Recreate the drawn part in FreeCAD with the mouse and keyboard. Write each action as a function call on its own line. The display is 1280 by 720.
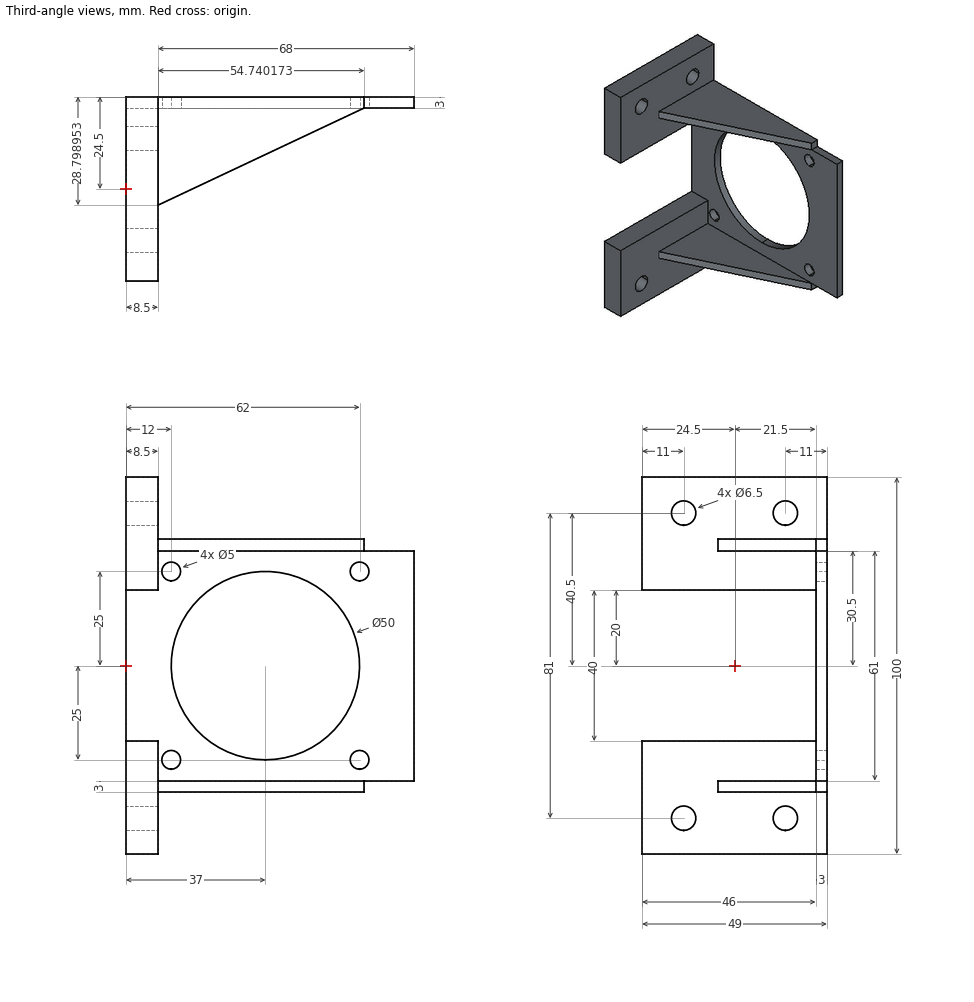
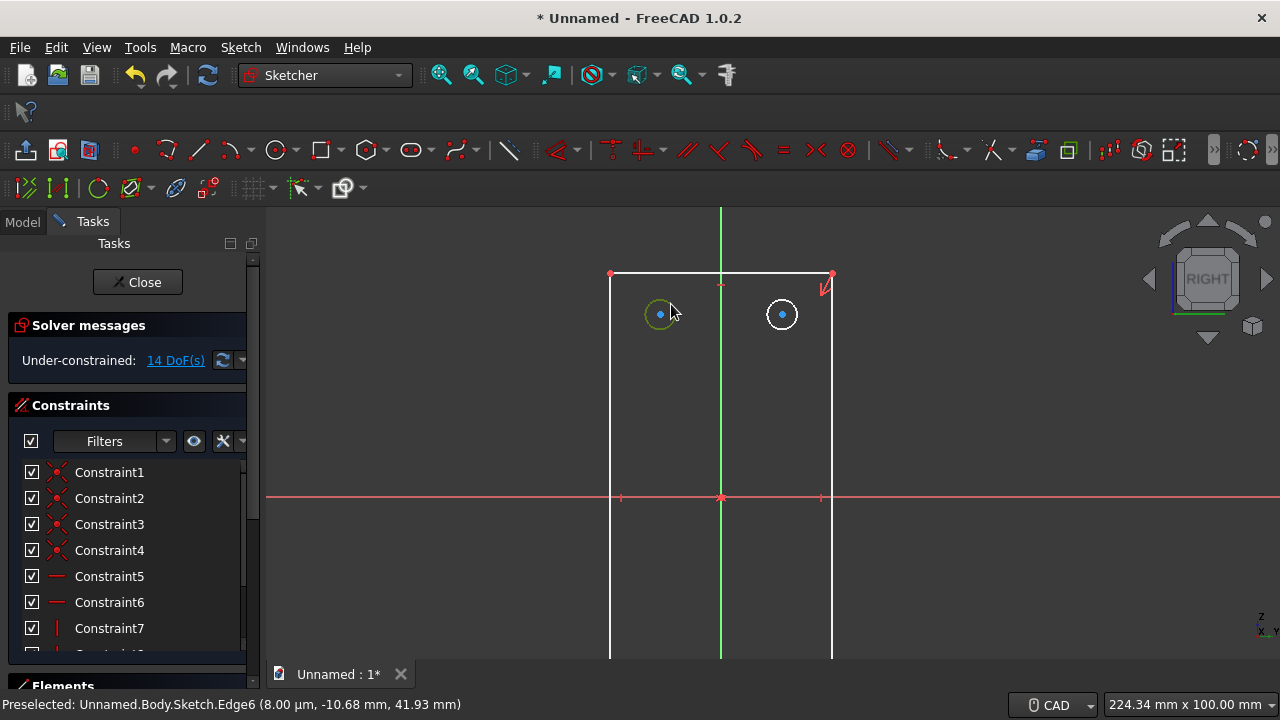
scroll(670, 303, down, 2)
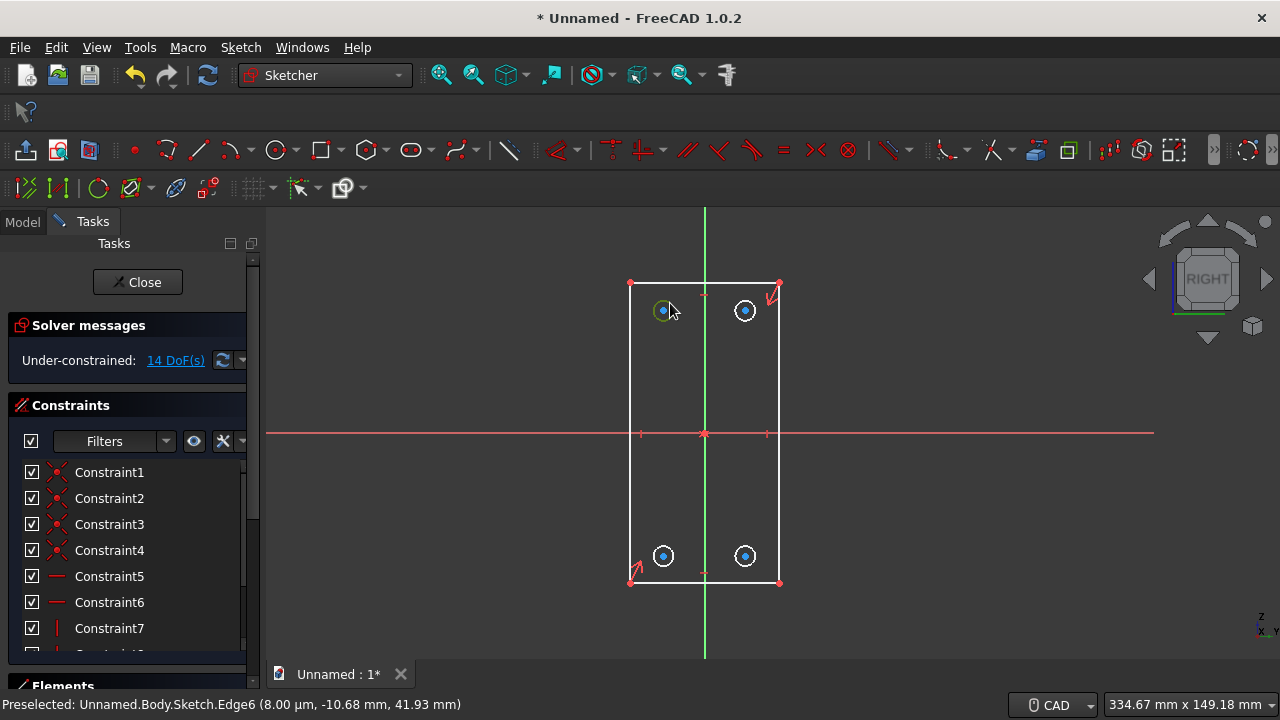
scroll(670, 549, up, 2)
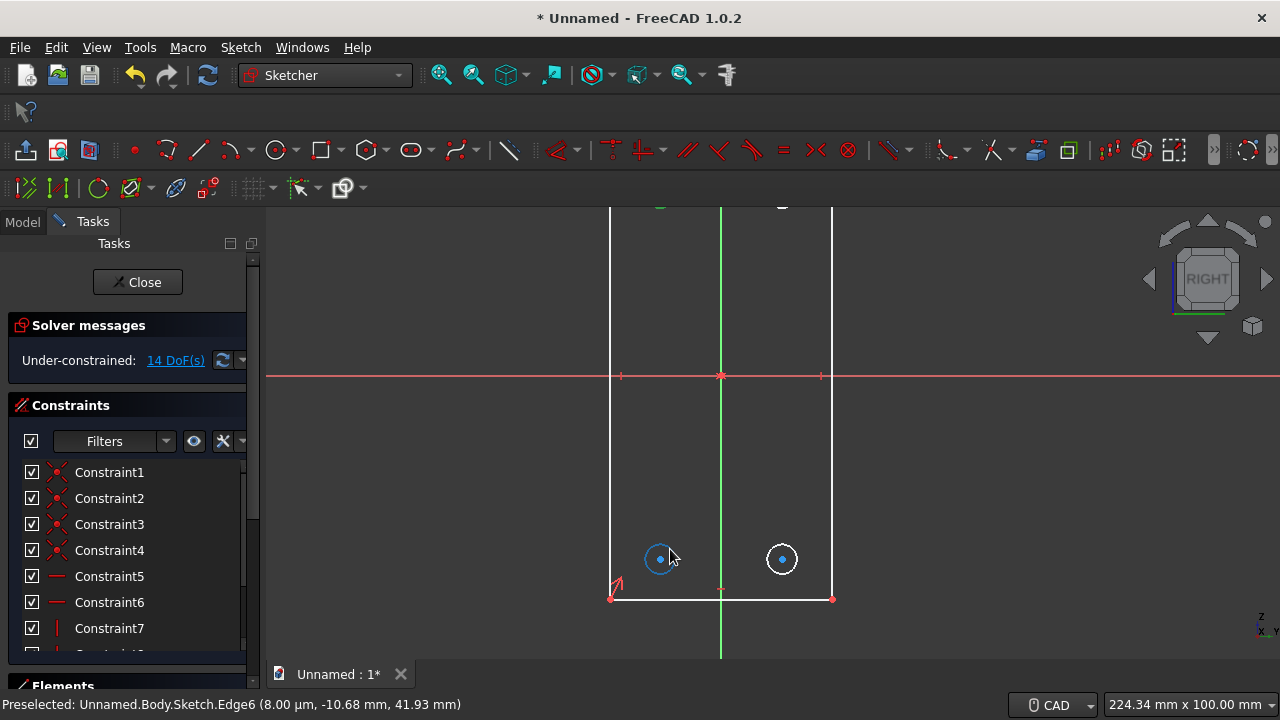
click(671, 549)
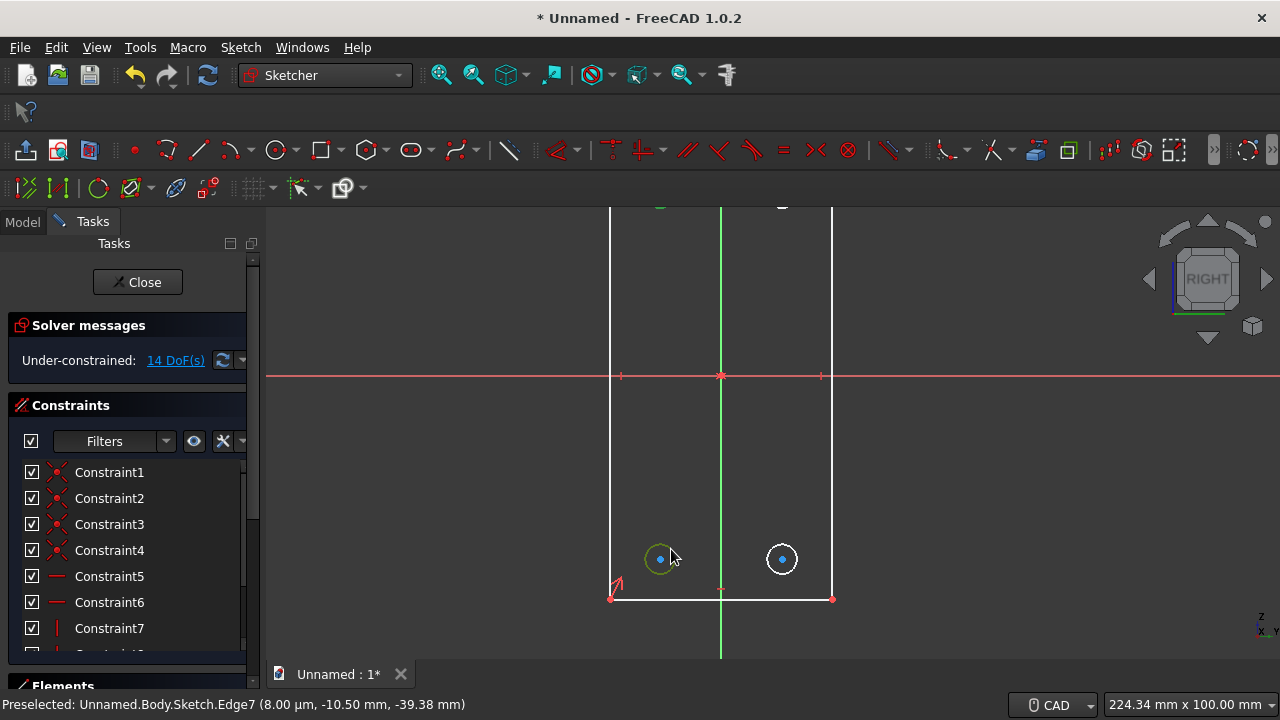
scroll(670, 549, down, 2)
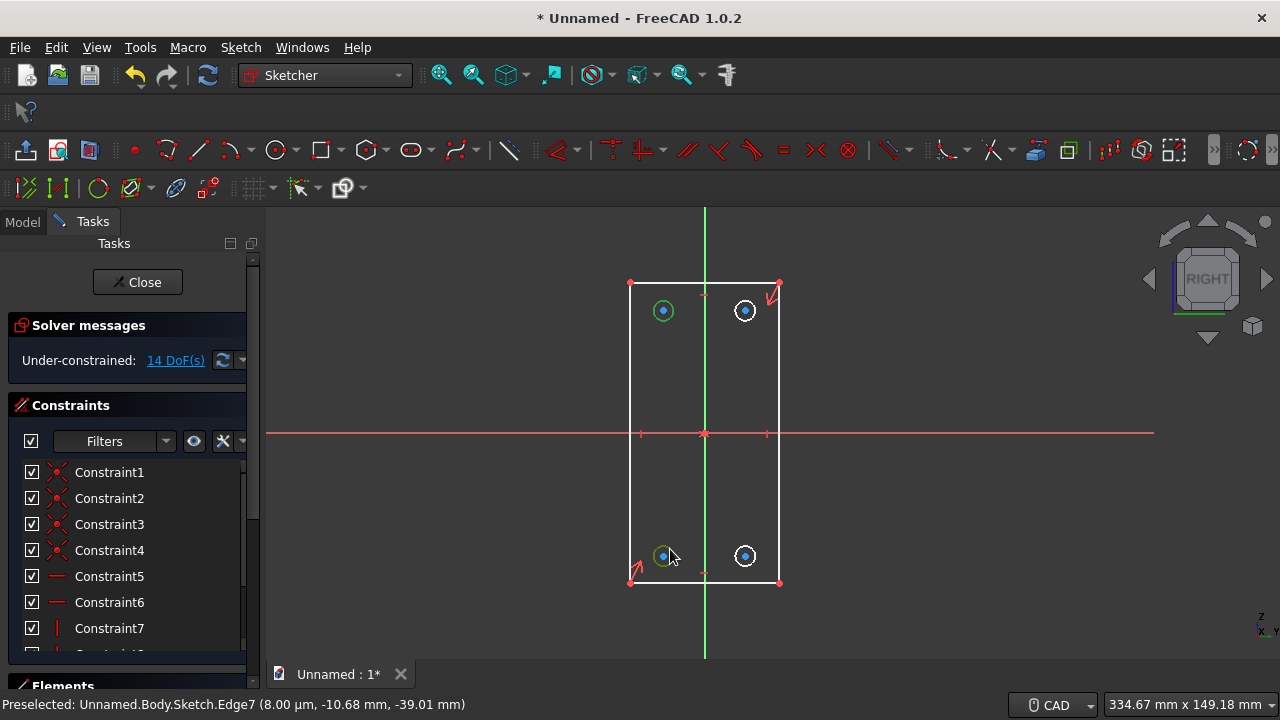
scroll(752, 304, up, 2)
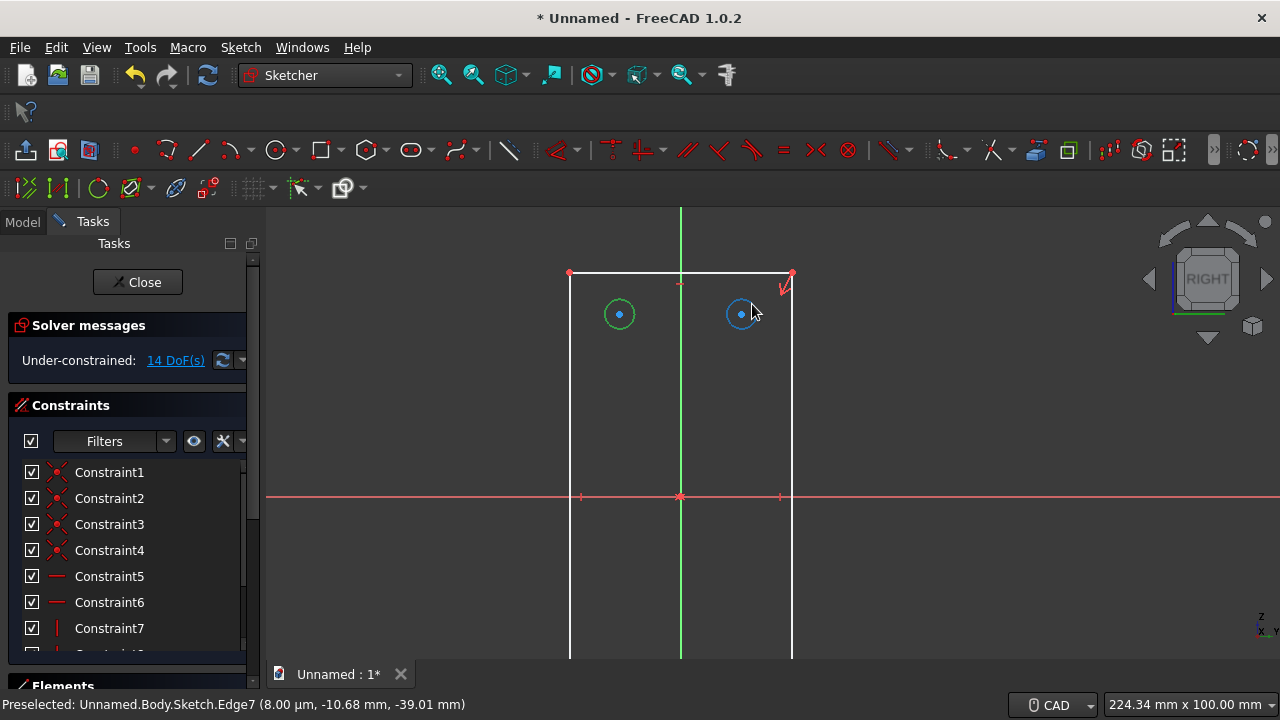
click(752, 304)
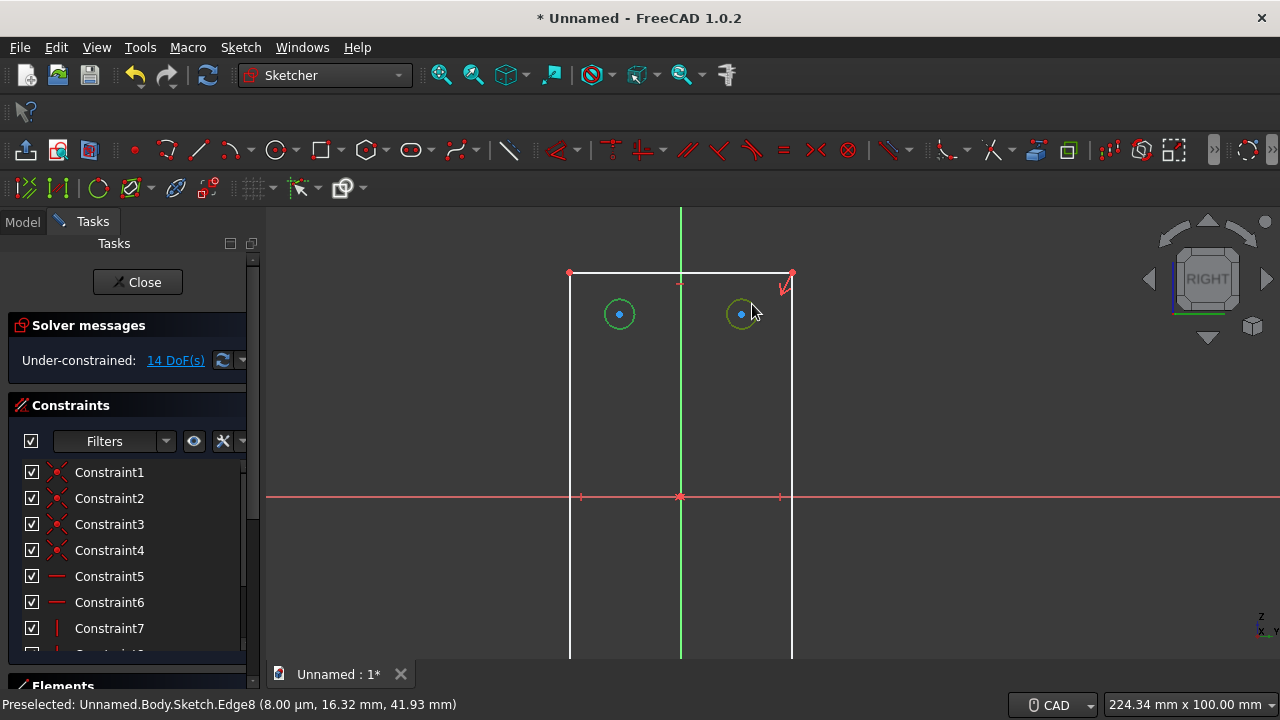
scroll(752, 304, down, 2)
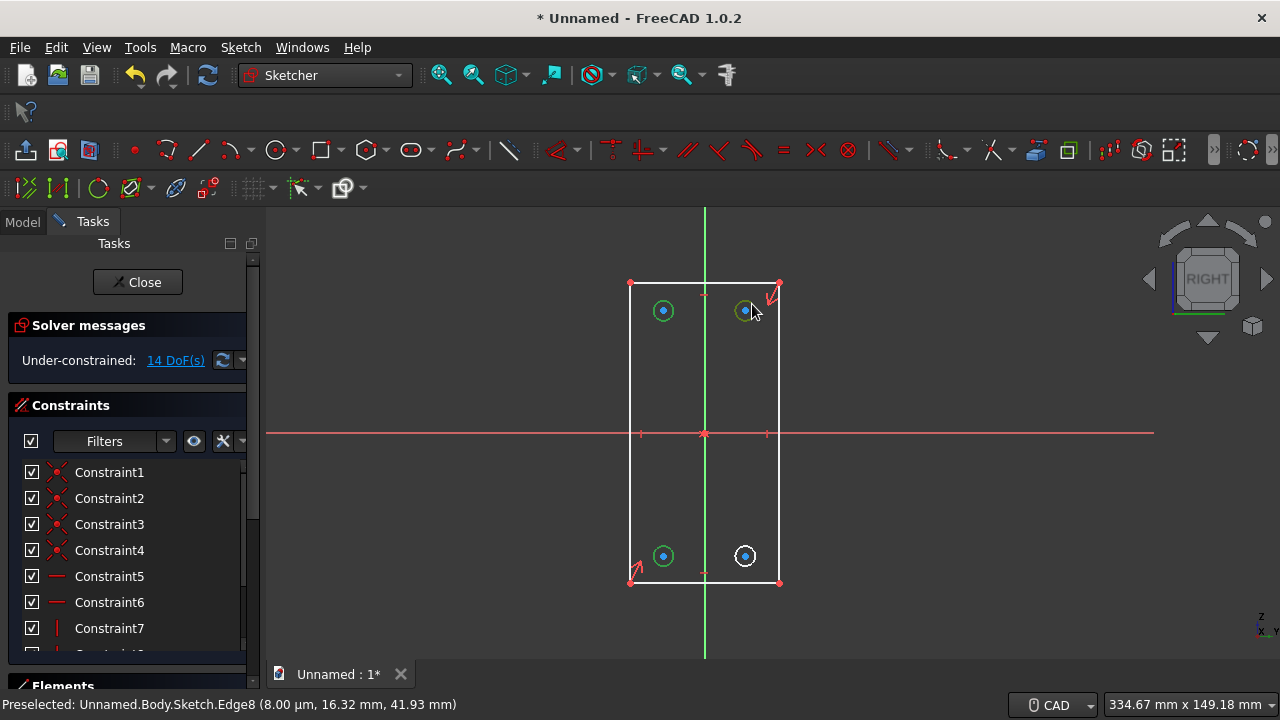
scroll(752, 549, up, 2)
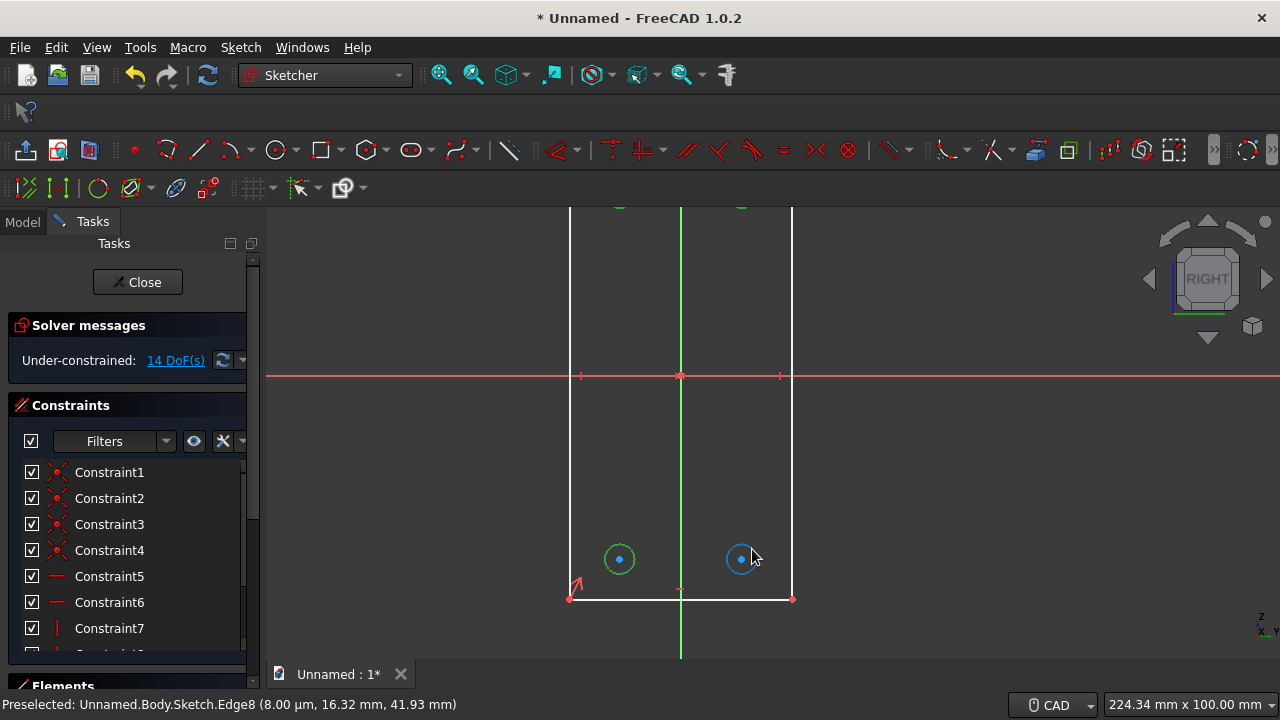
click(752, 549)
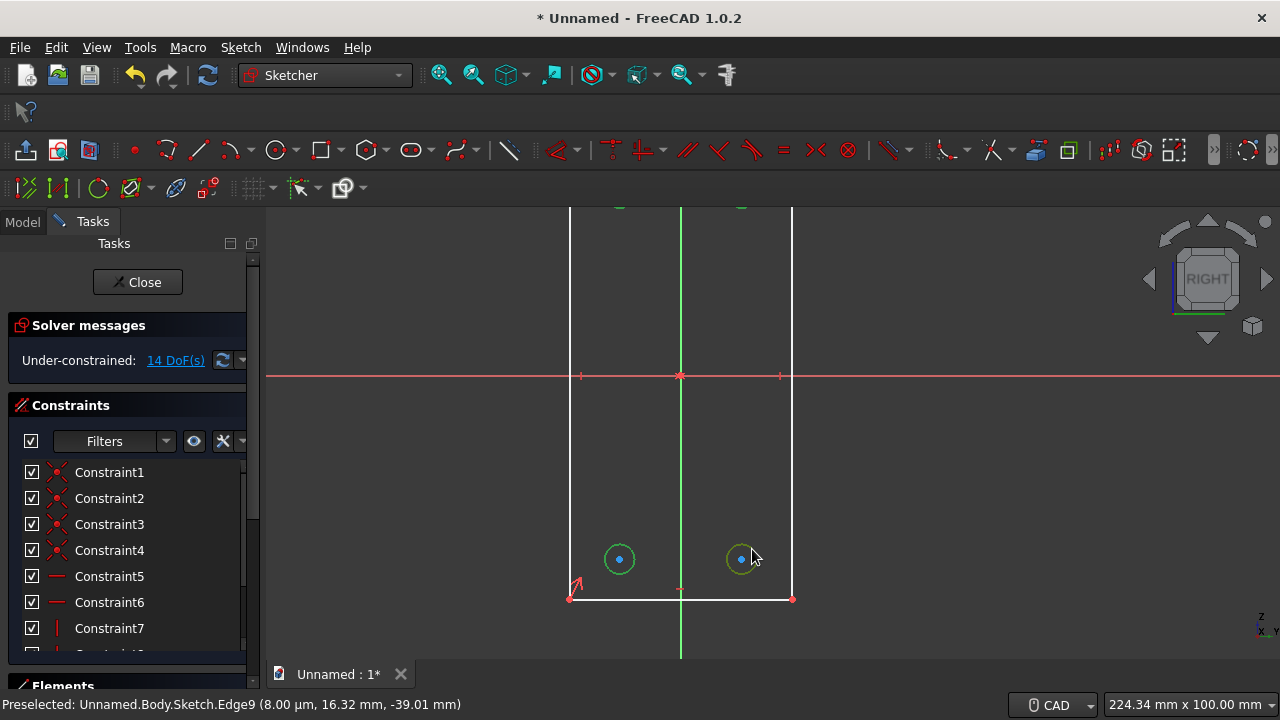
click(784, 150)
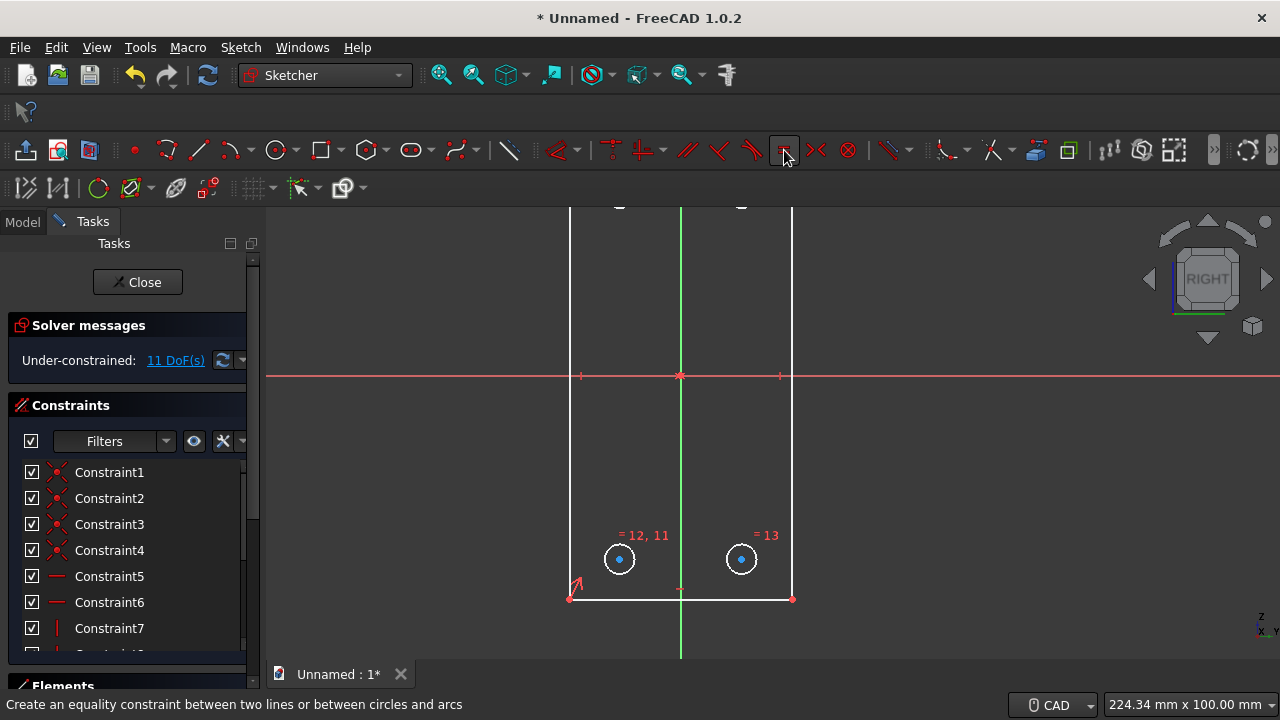
scroll(752, 549, down, 2)